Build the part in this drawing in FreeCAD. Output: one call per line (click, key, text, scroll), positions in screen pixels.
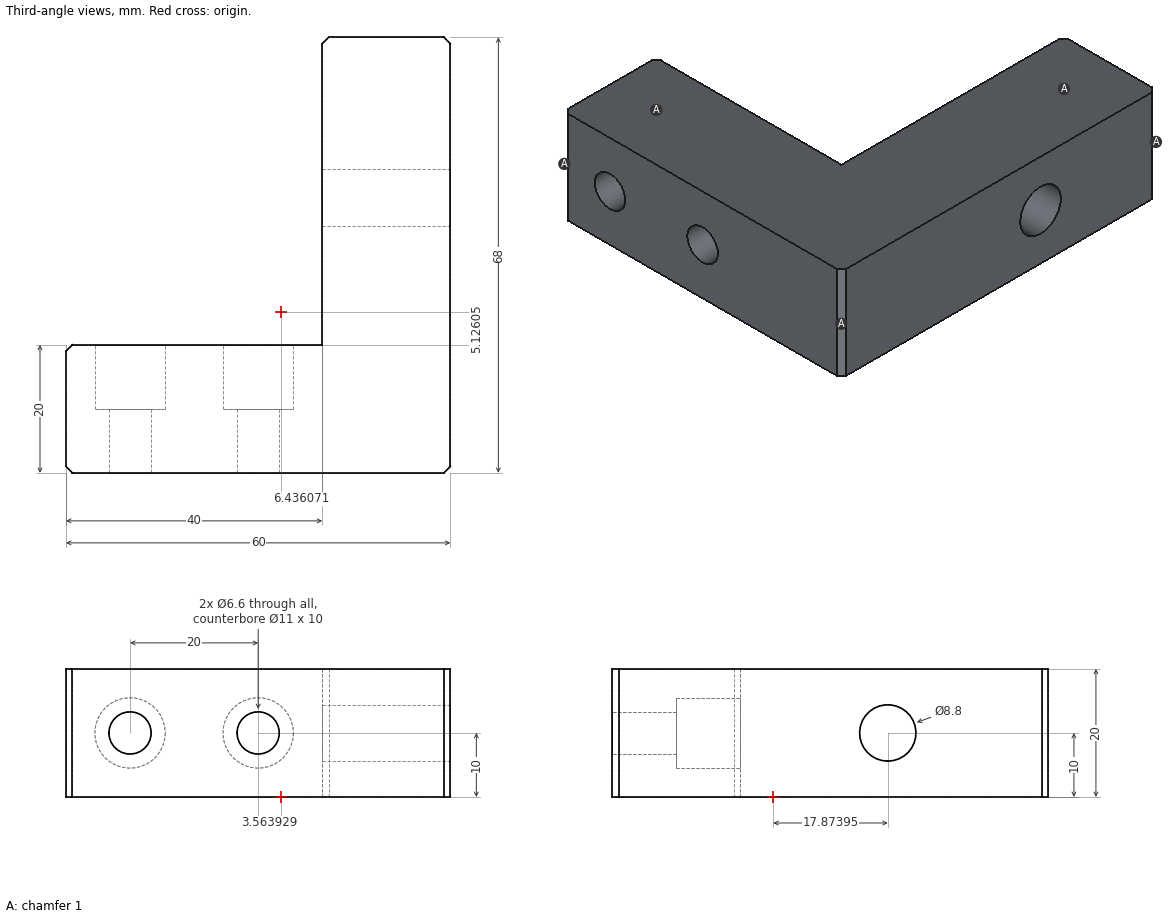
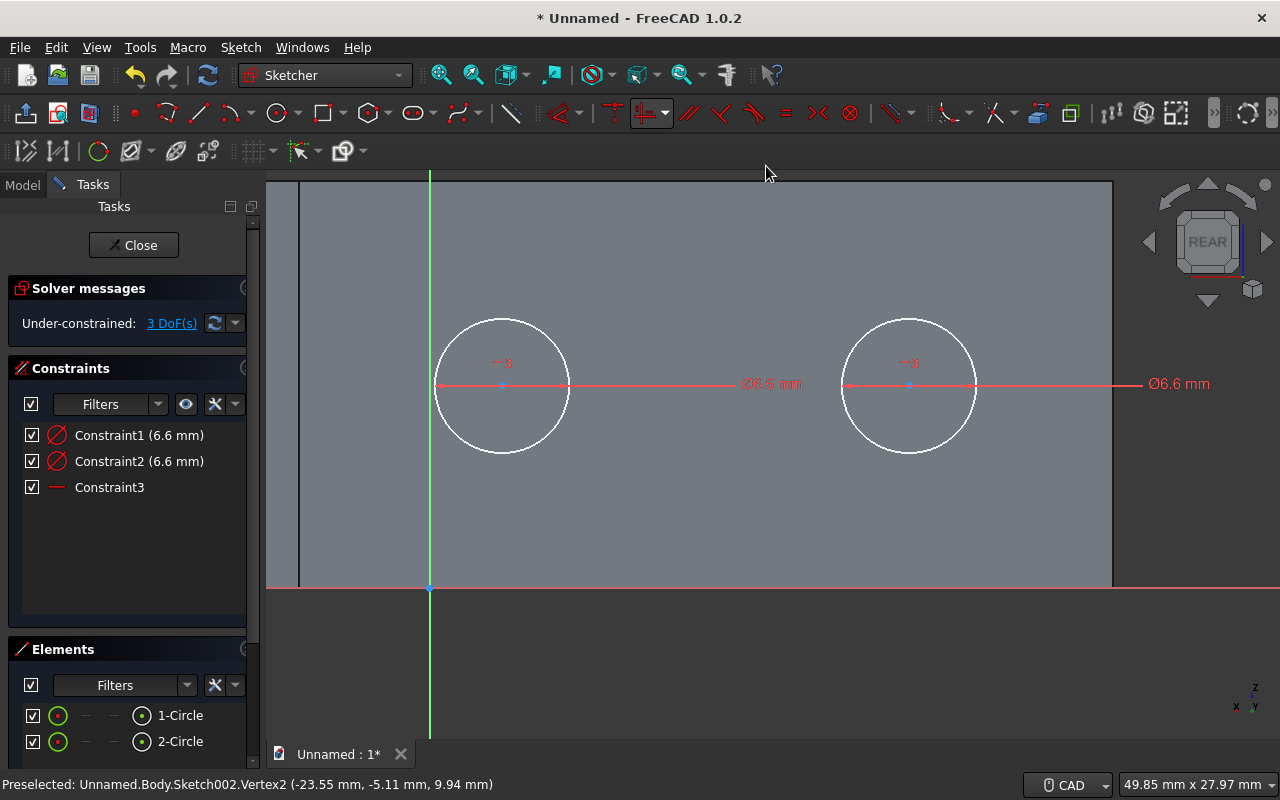
click(502, 386)
click(396, 487)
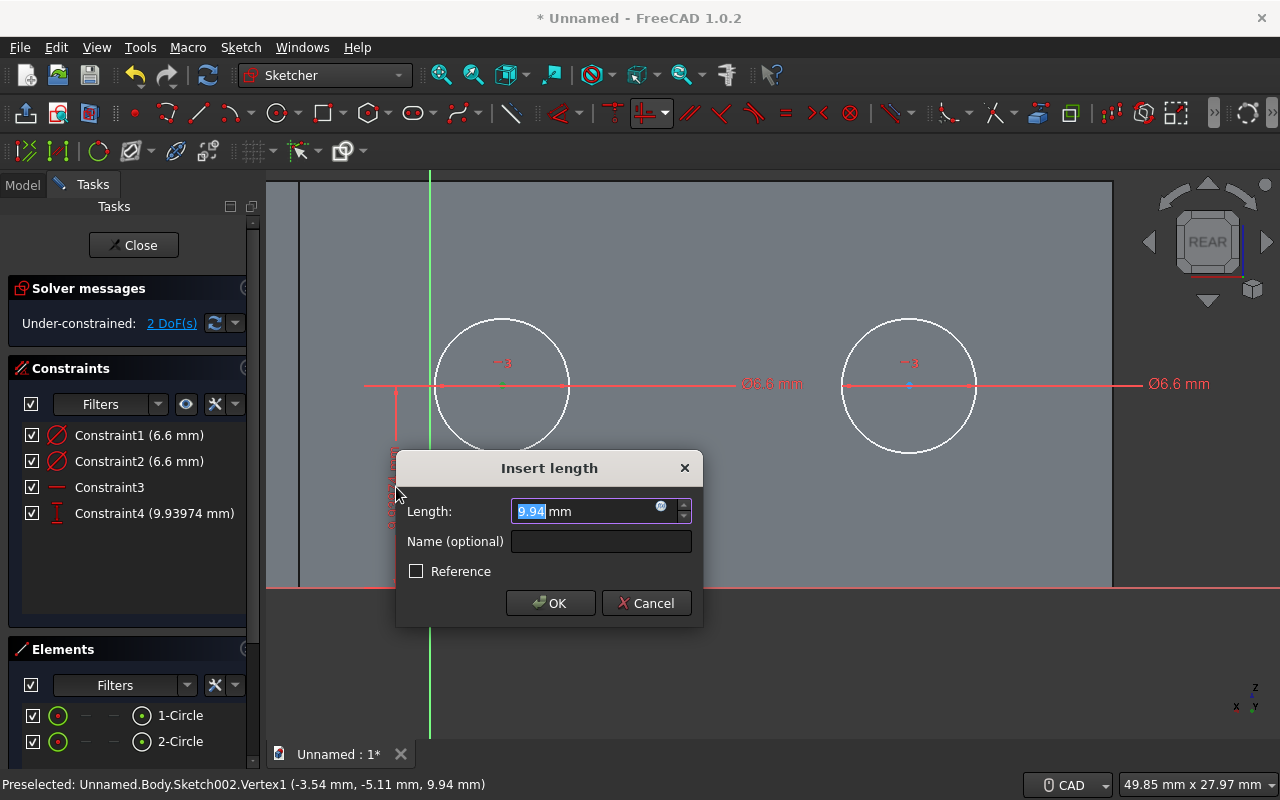
text(10)
key(Return)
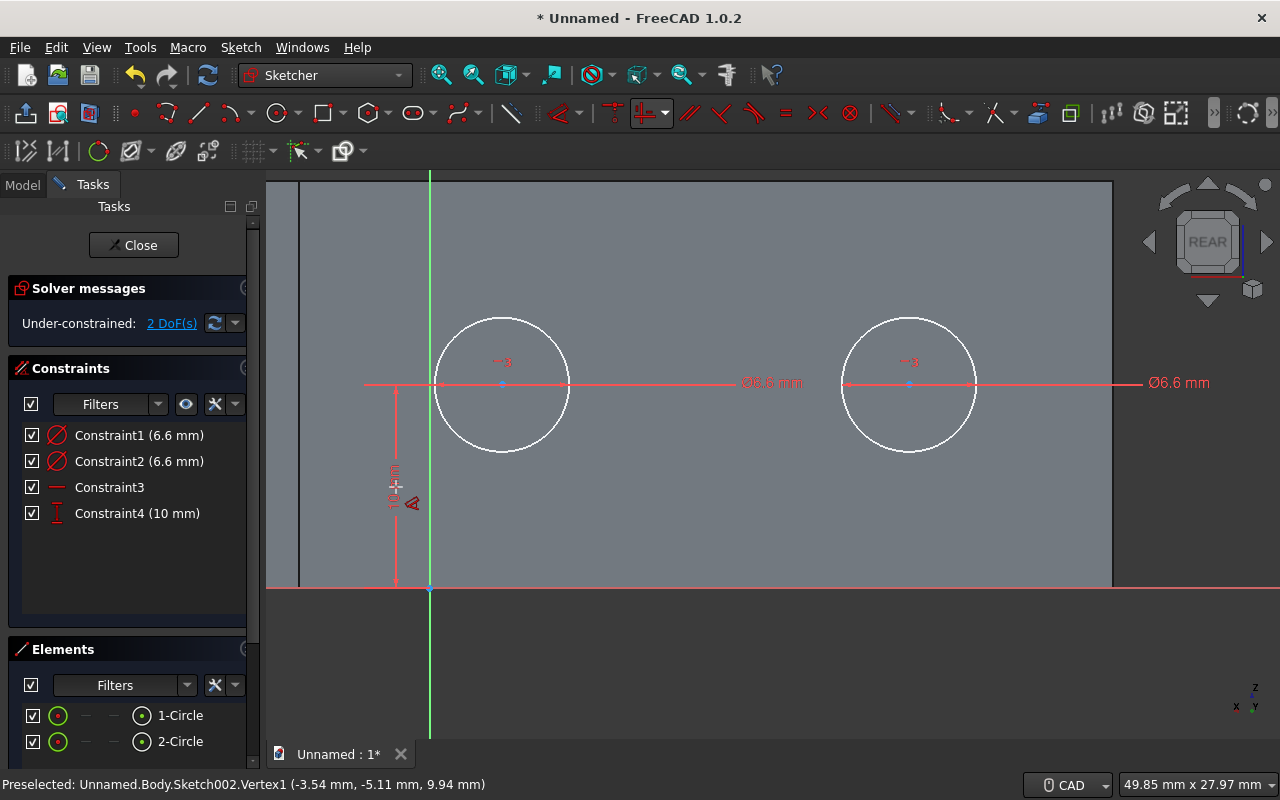
click(502, 385)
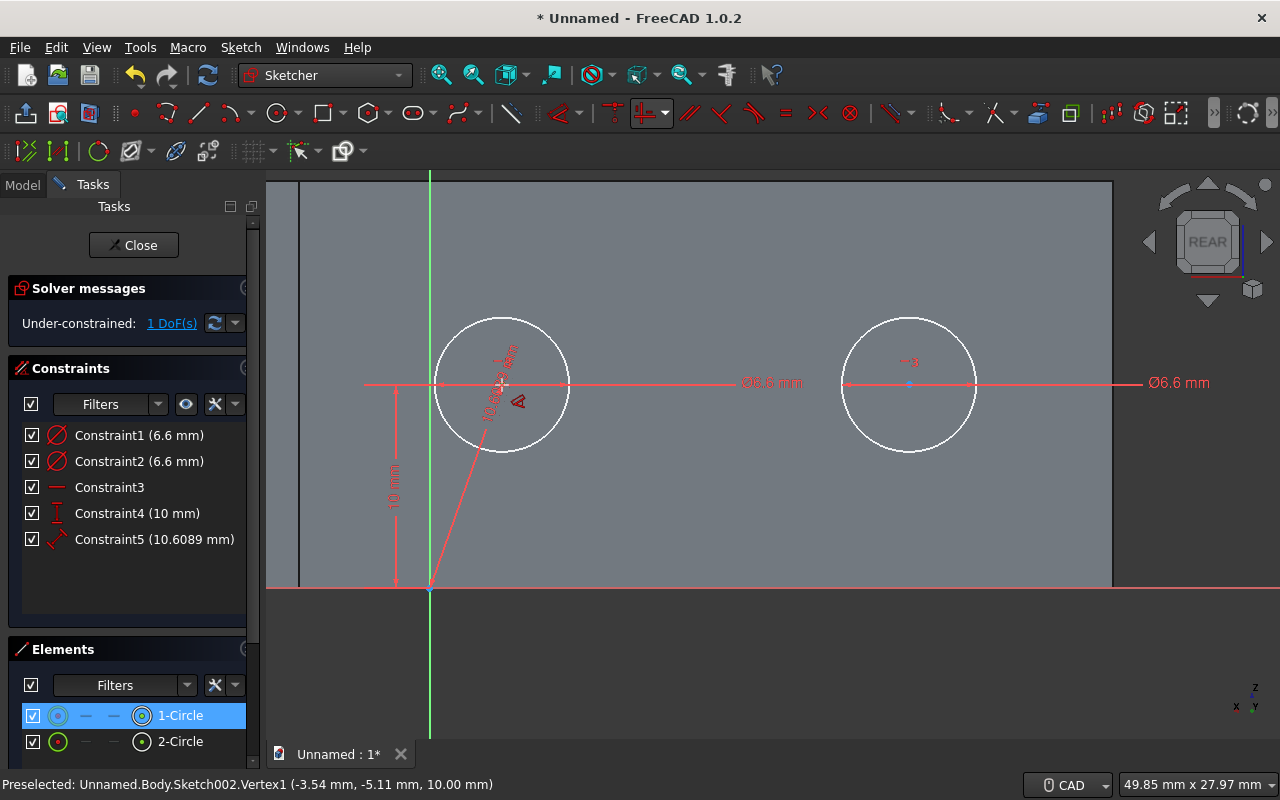
click(909, 385)
click(706, 351)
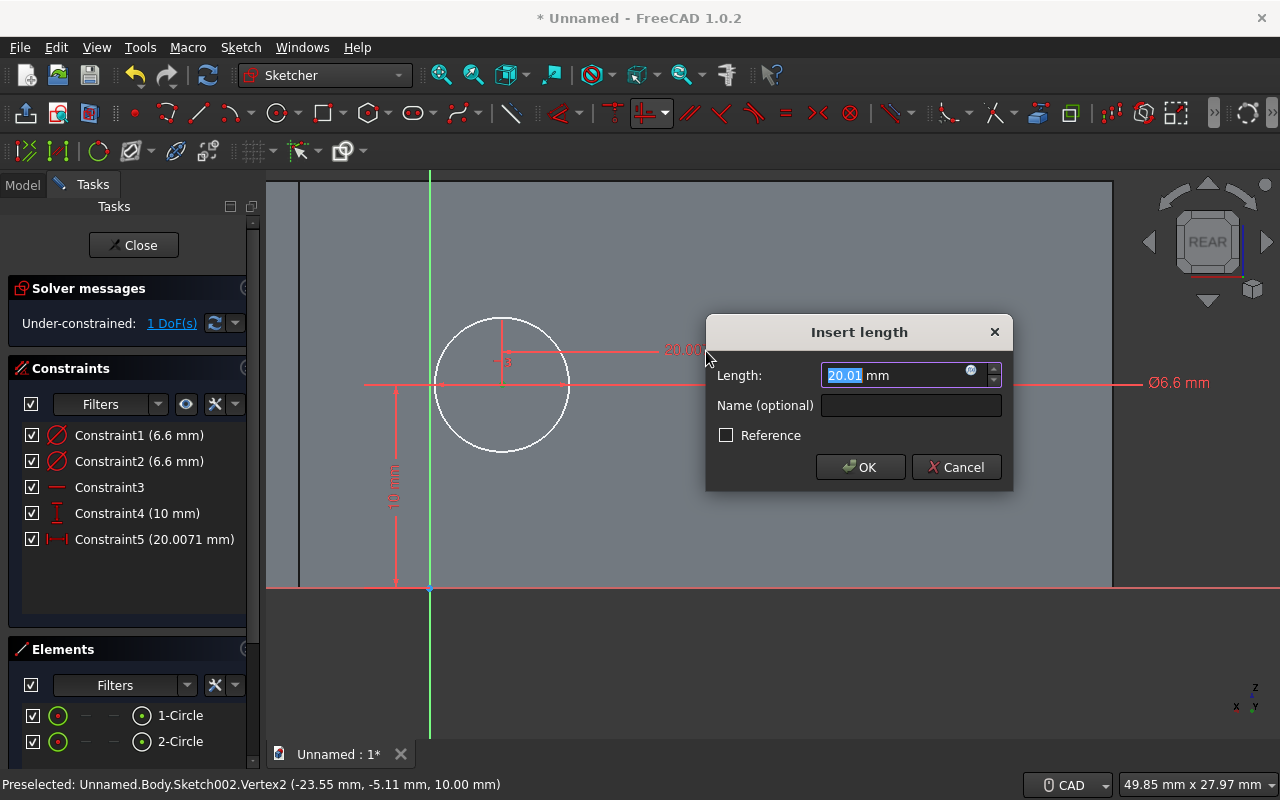
text(20)
key(Return)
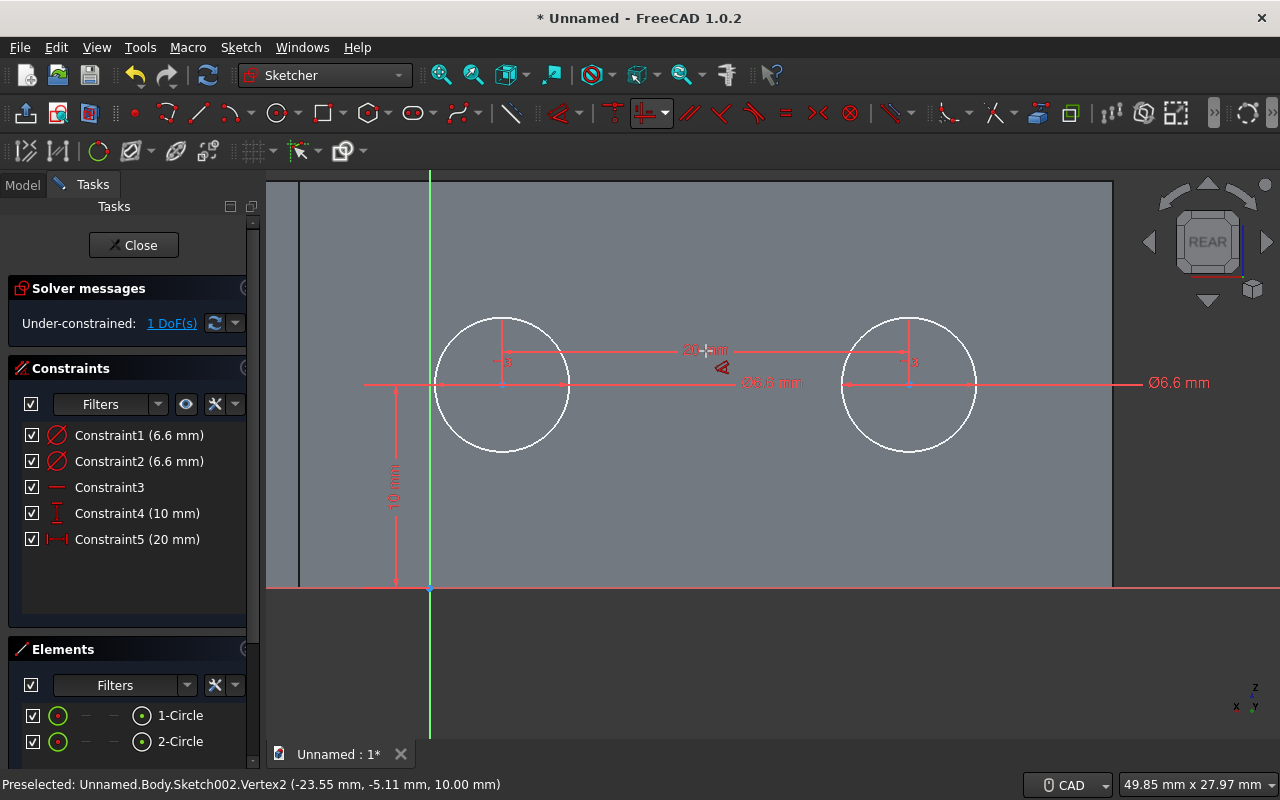
click(502, 385)
click(466, 622)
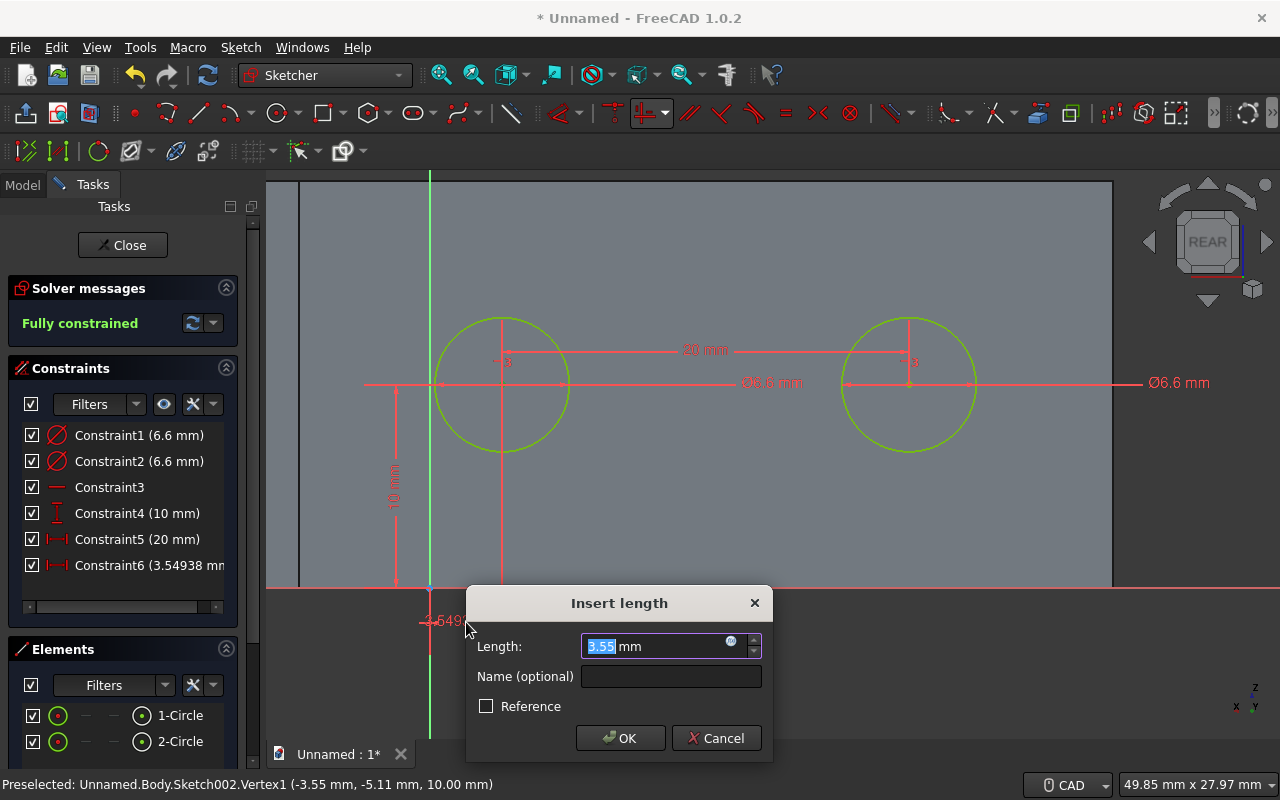
text(3.563929)
key(Return)
key(Escape)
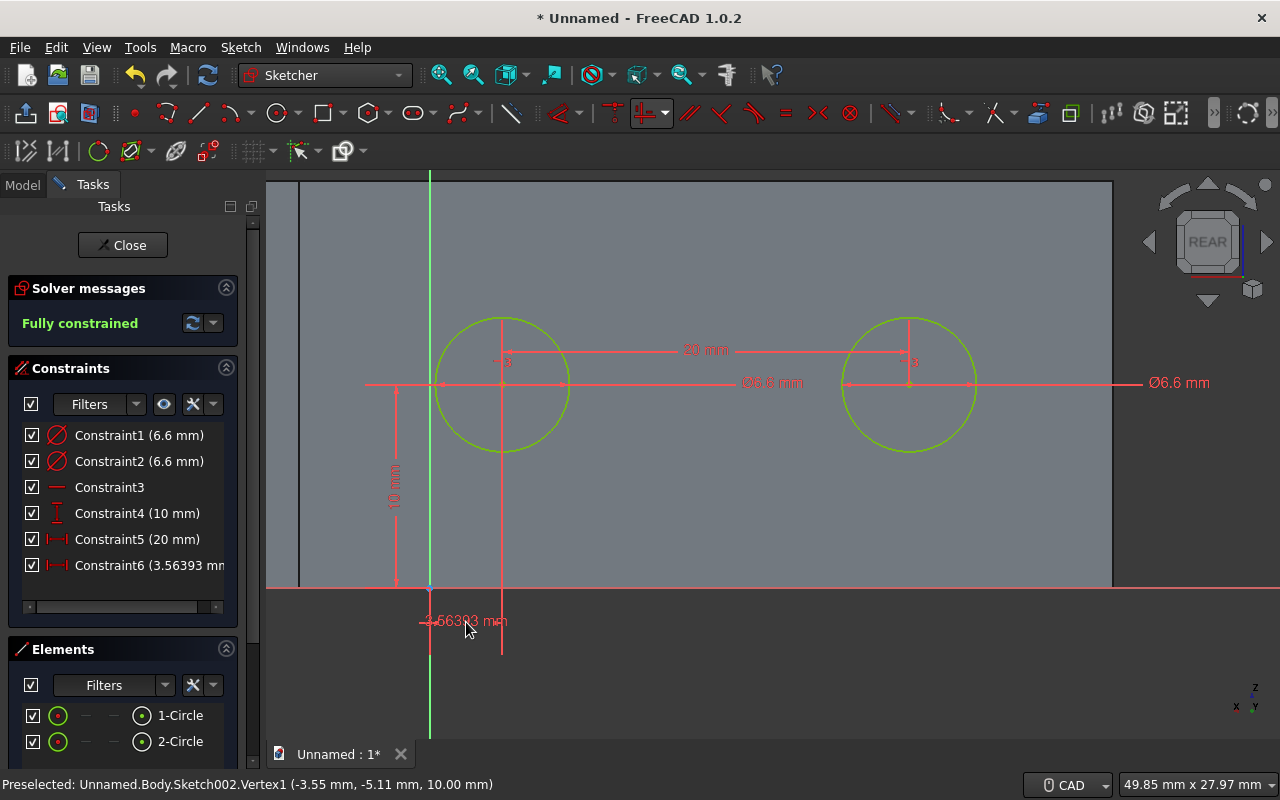
click(123, 245)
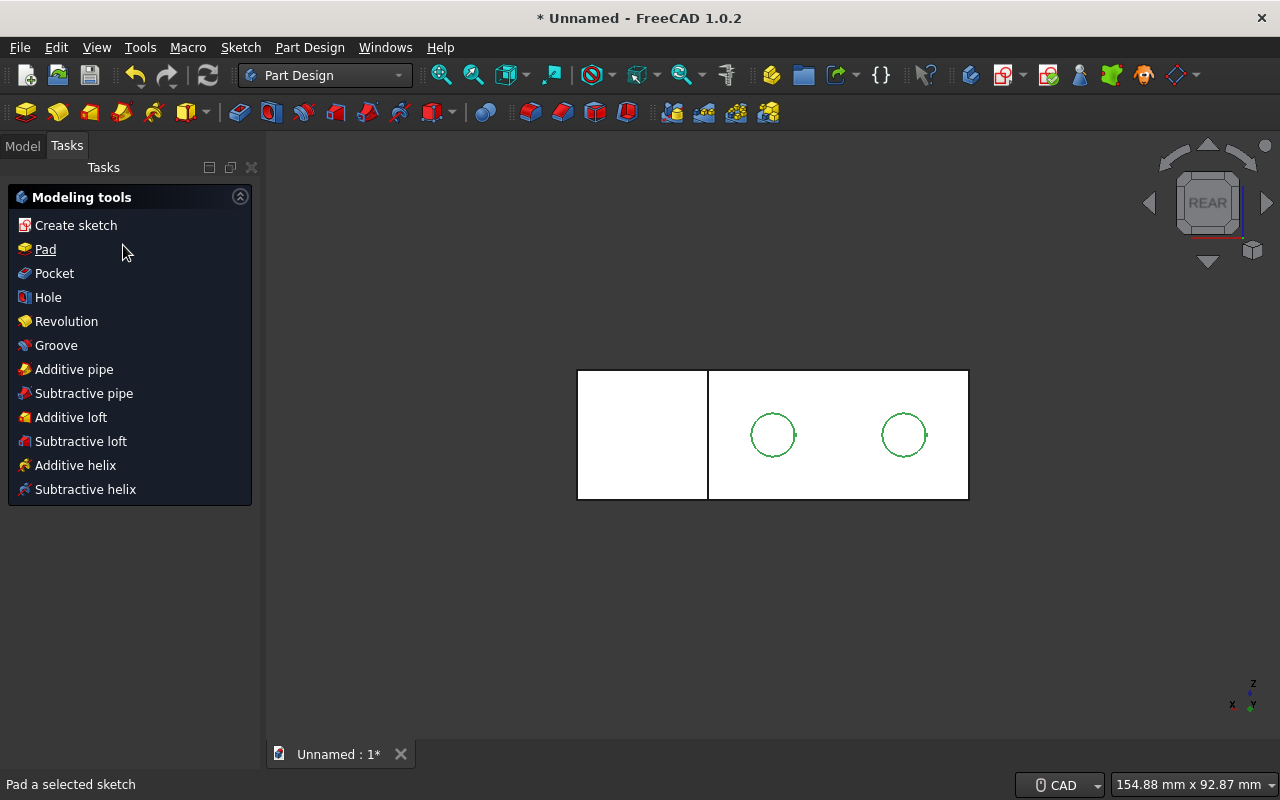
click(272, 112)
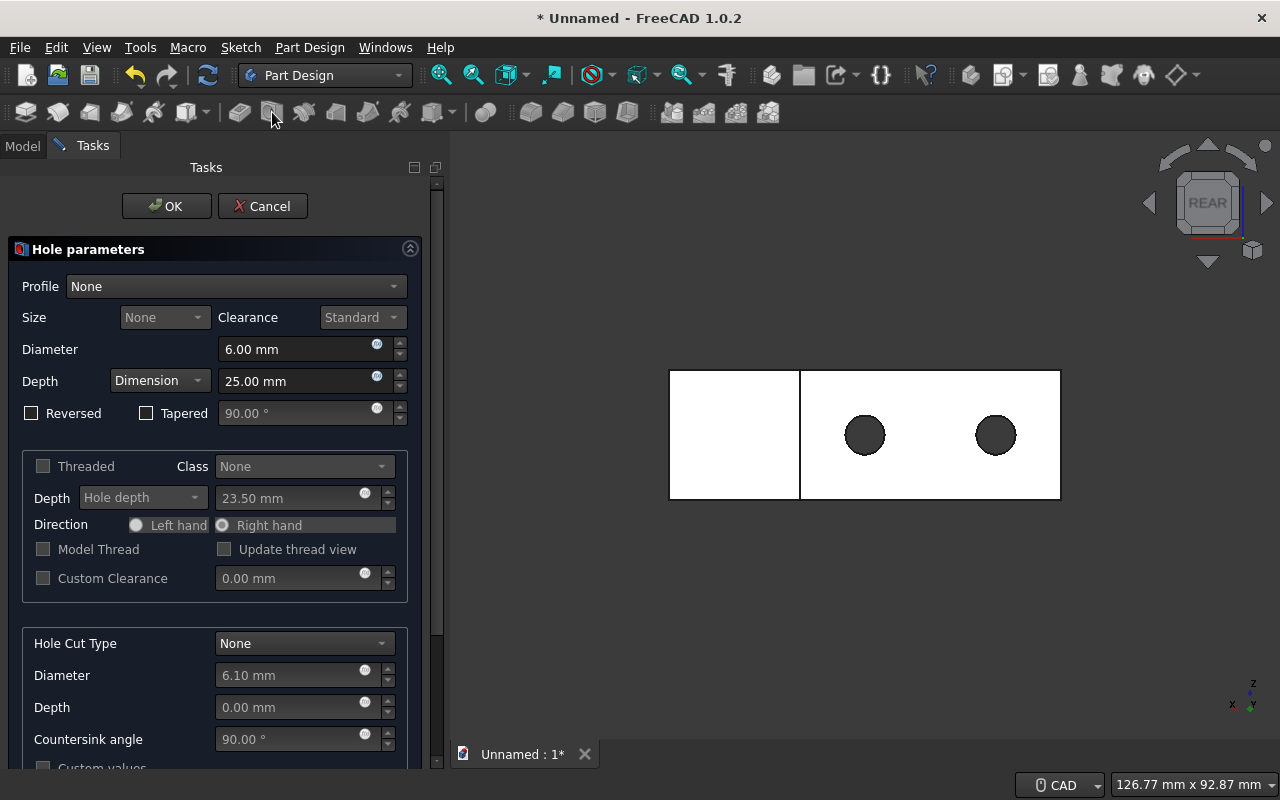
triple_click(305, 349)